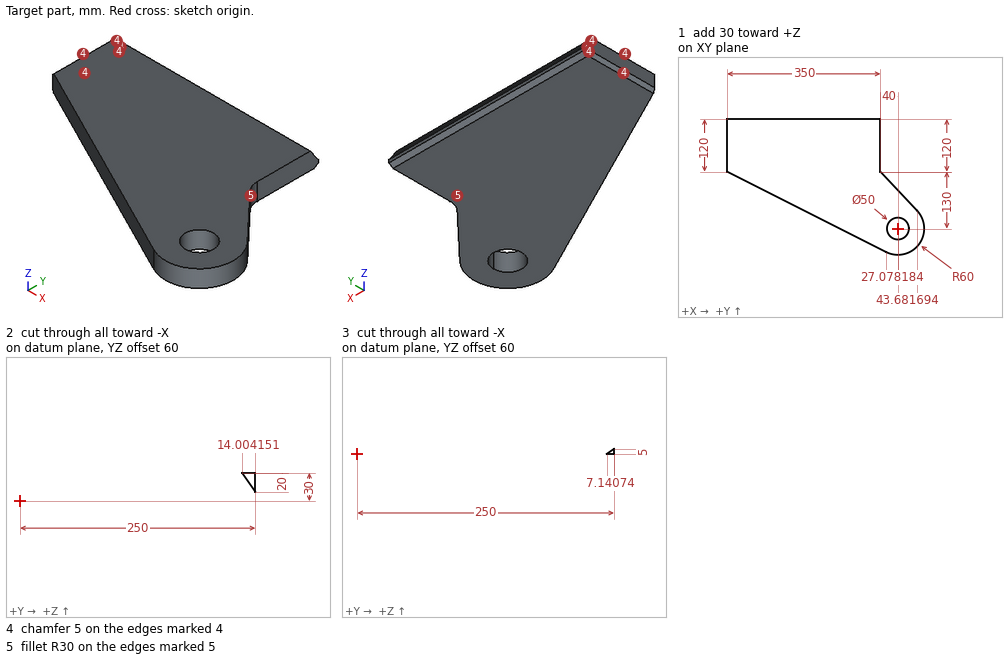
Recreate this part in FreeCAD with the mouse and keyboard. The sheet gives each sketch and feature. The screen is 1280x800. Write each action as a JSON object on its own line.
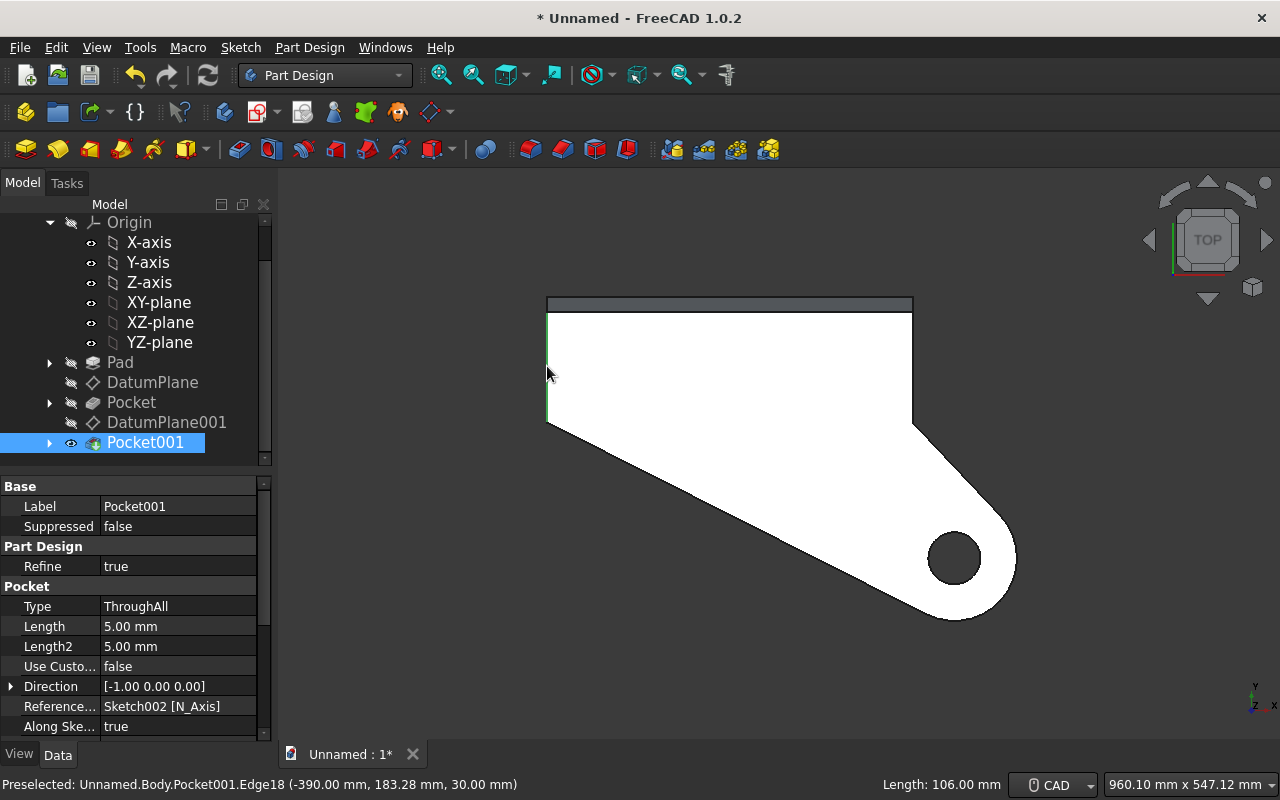
{"action": "left_click", "coordinate": [547, 304], "text": "ctrl"}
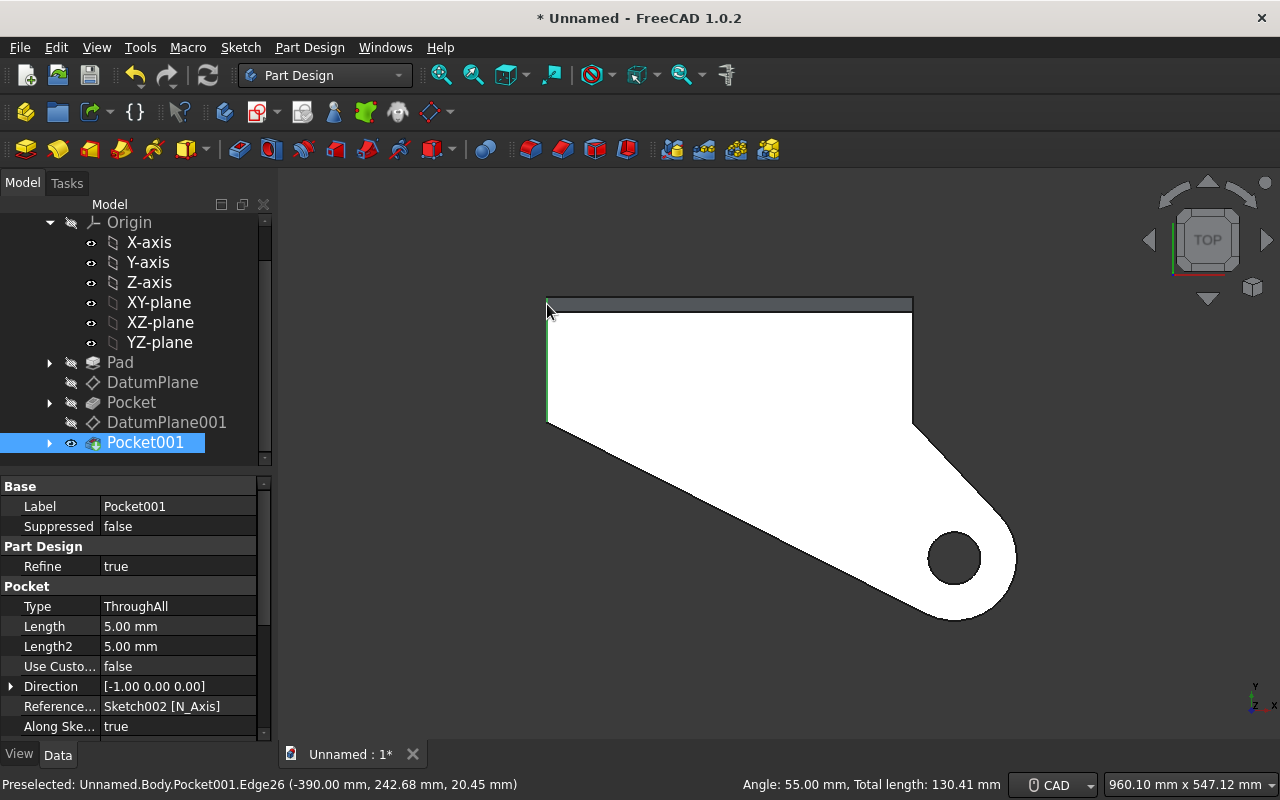
{"action": "scroll", "coordinate": [547, 296], "scroll_direction": "up", "scroll_amount": 11}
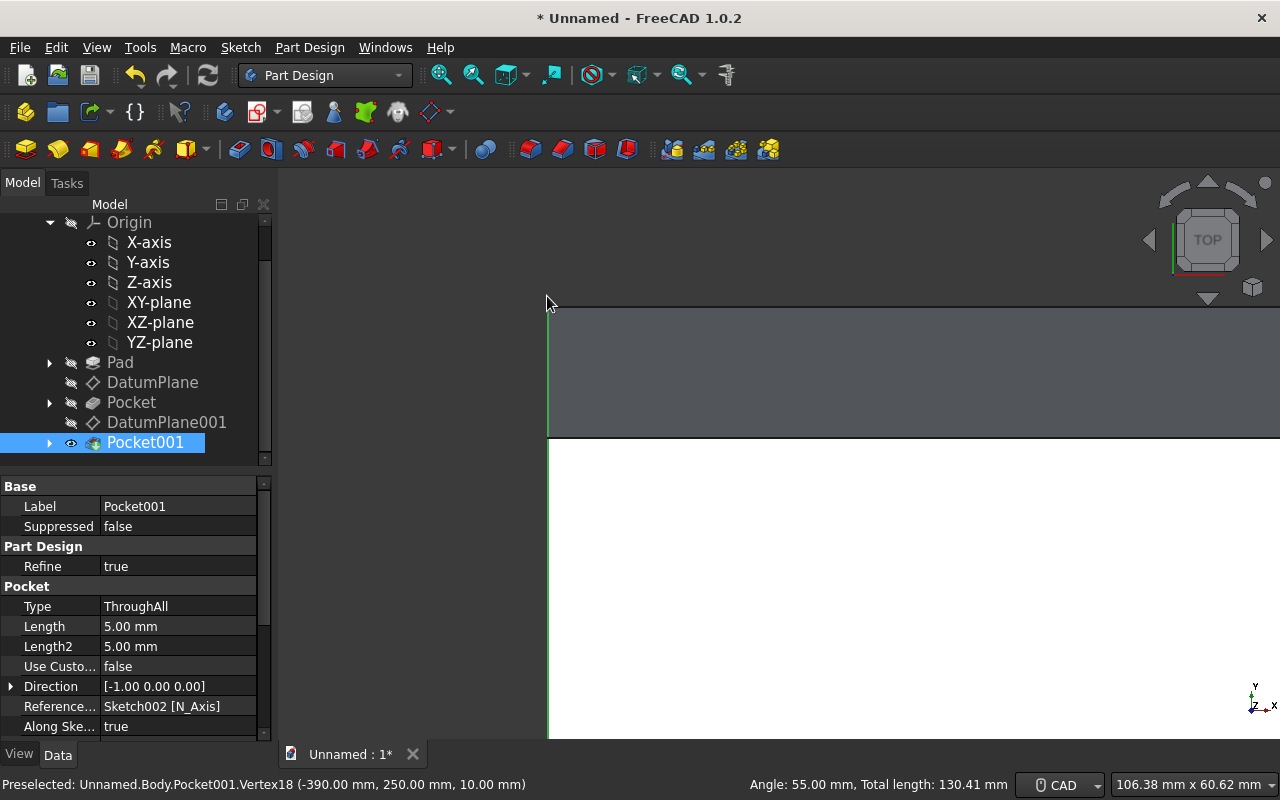
{"action": "key", "text": "v f"}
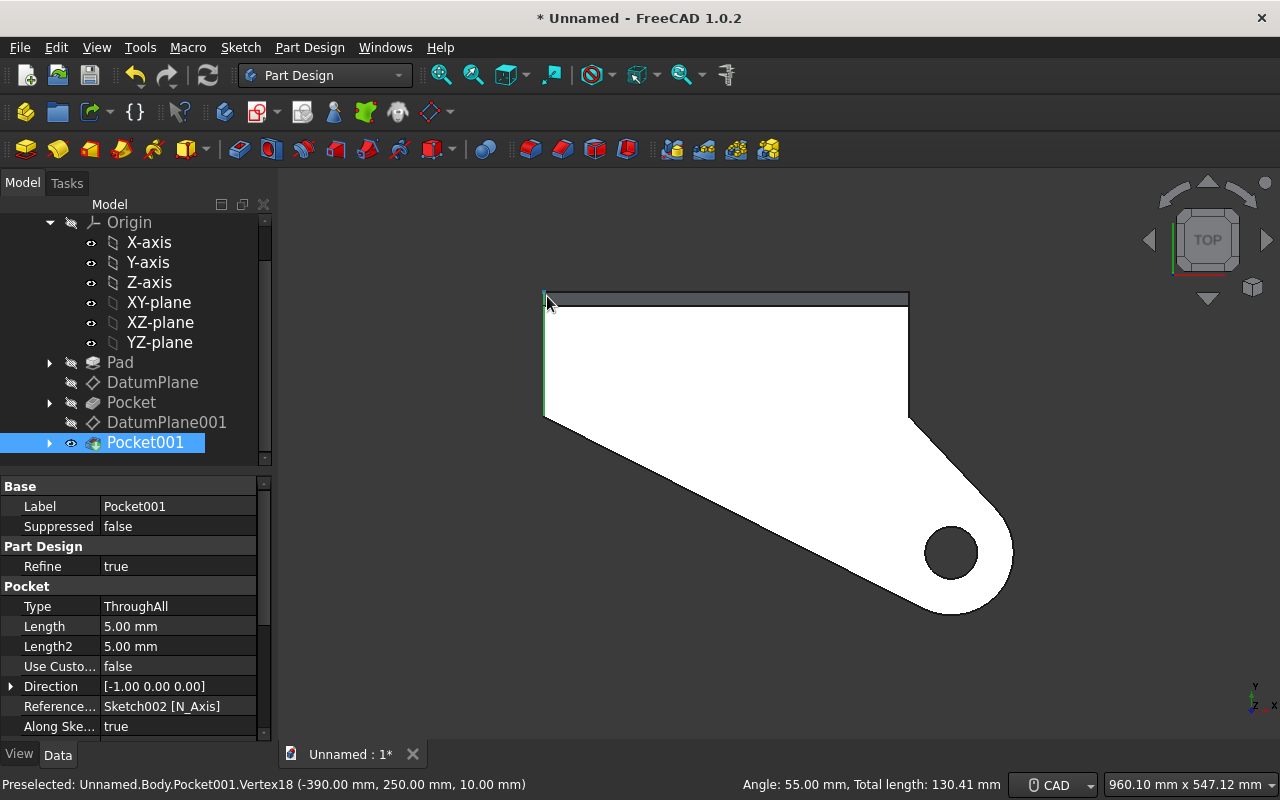
{"action": "key", "text": "1"}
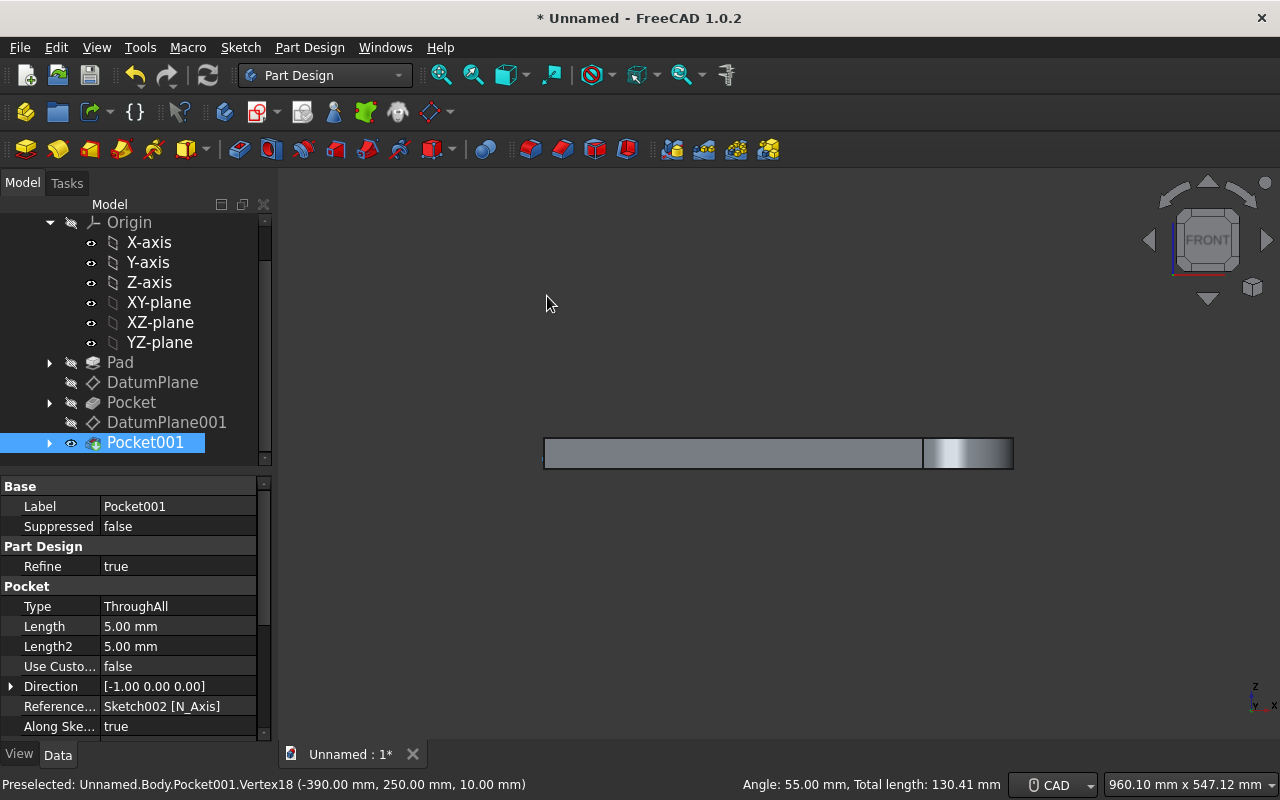
{"action": "scroll", "coordinate": [544, 460], "scroll_direction": "up", "scroll_amount": 11}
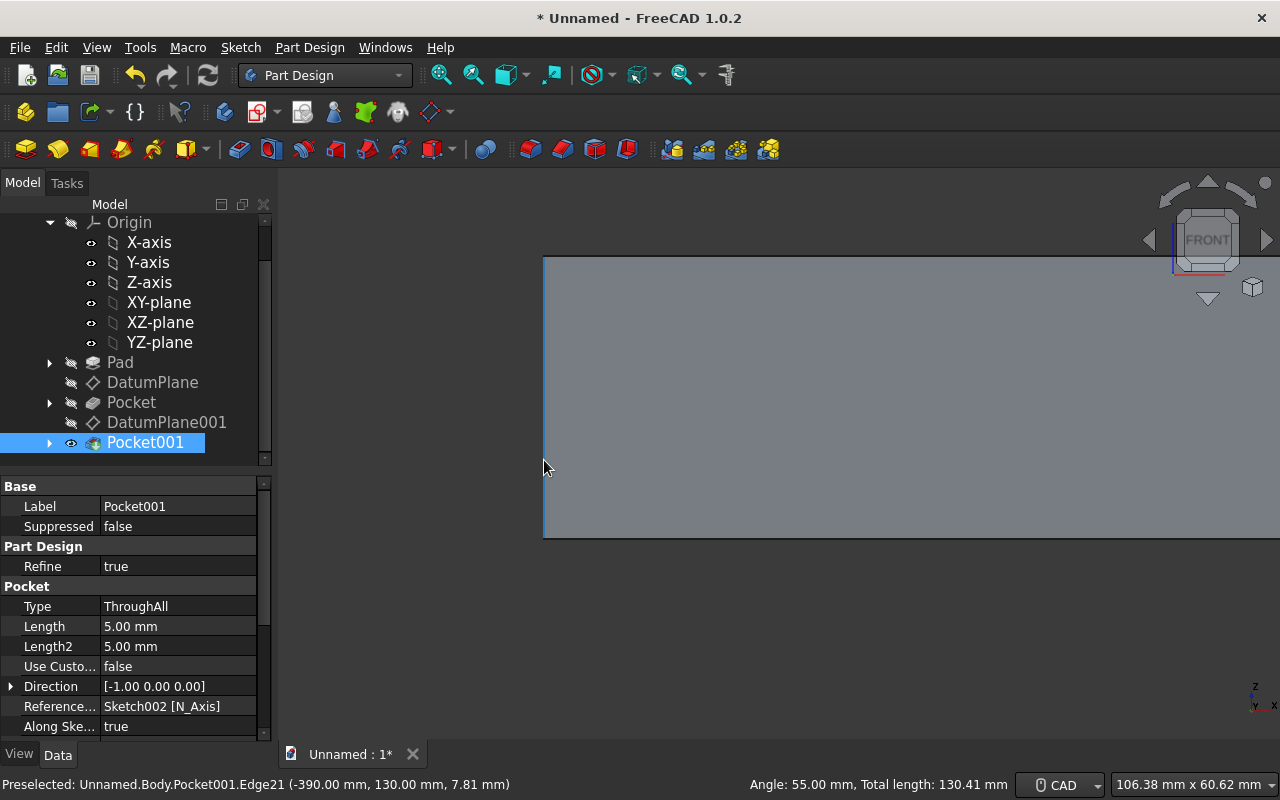
{"action": "key", "text": "v f"}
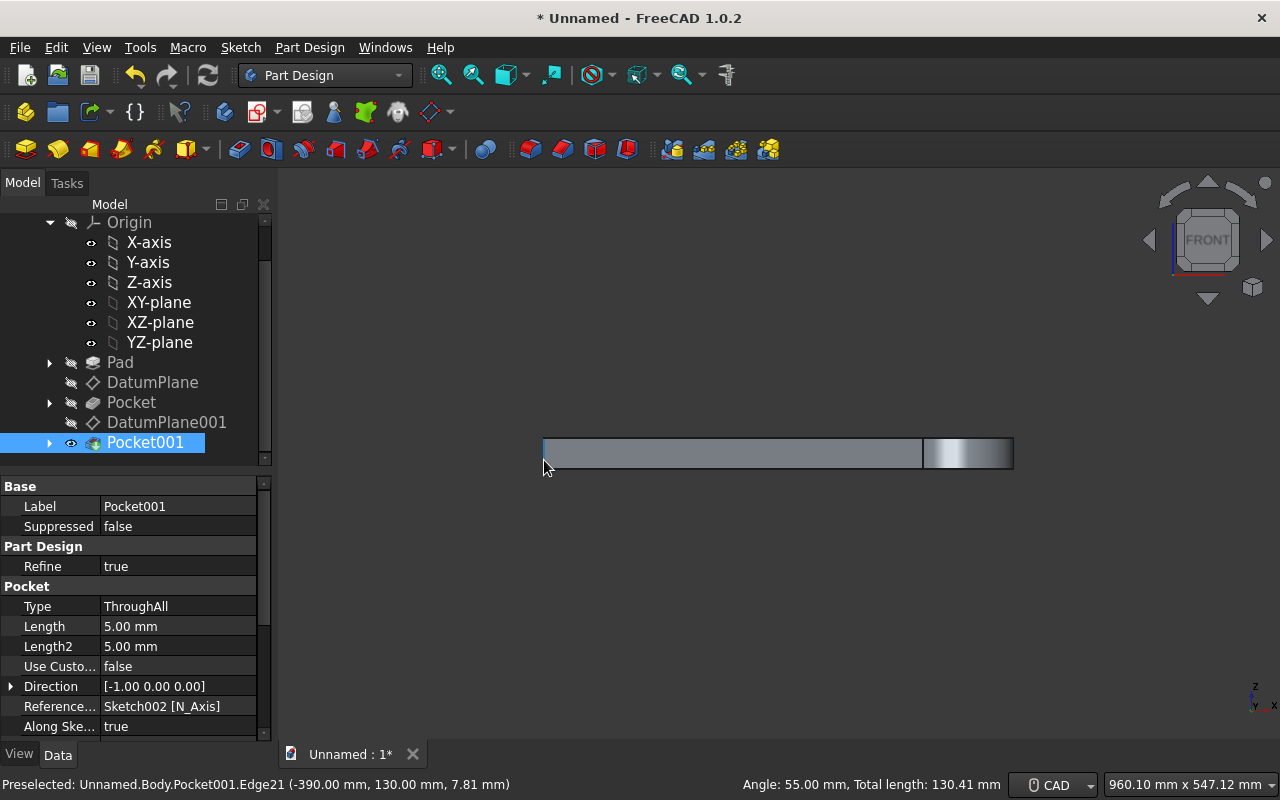
{"action": "key", "text": "3"}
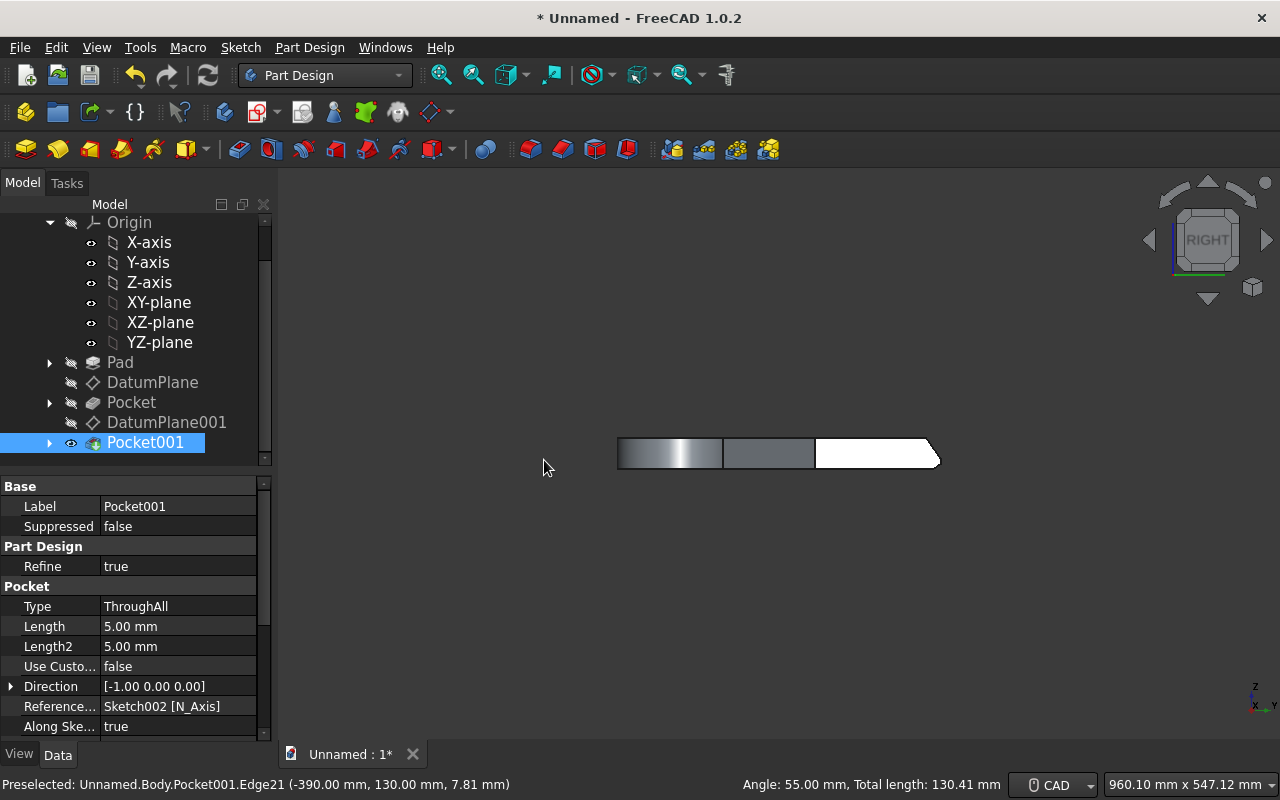
{"action": "key", "text": "v f"}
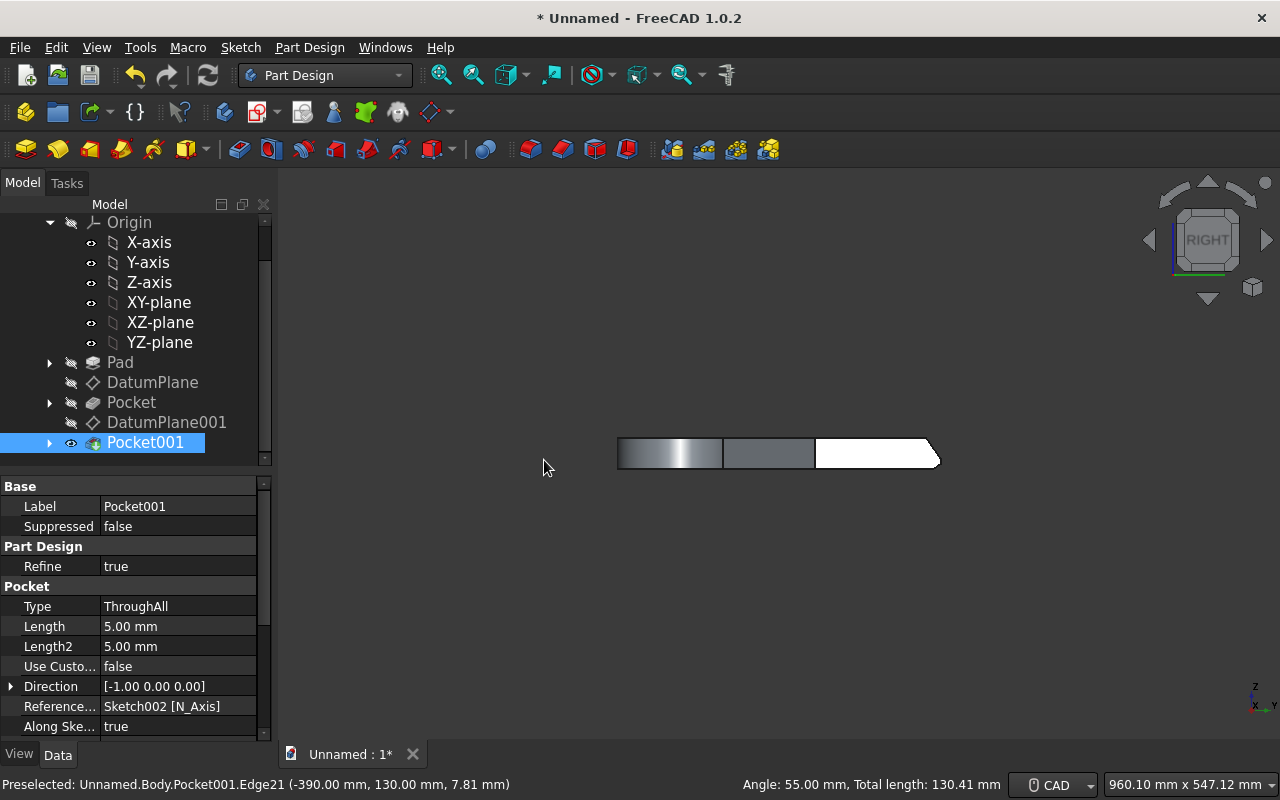
{"action": "scroll", "coordinate": [941, 460], "scroll_direction": "up", "scroll_amount": 11}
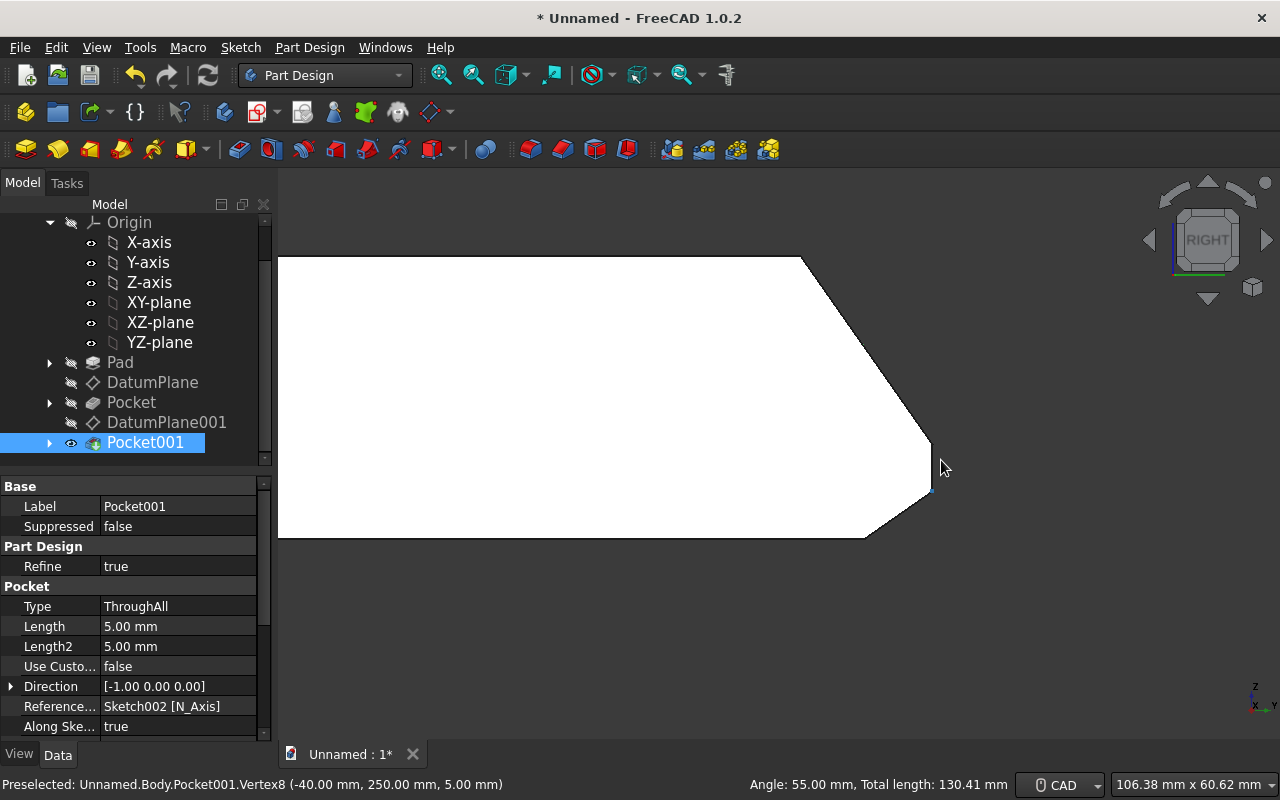
{"action": "key", "text": "v f"}